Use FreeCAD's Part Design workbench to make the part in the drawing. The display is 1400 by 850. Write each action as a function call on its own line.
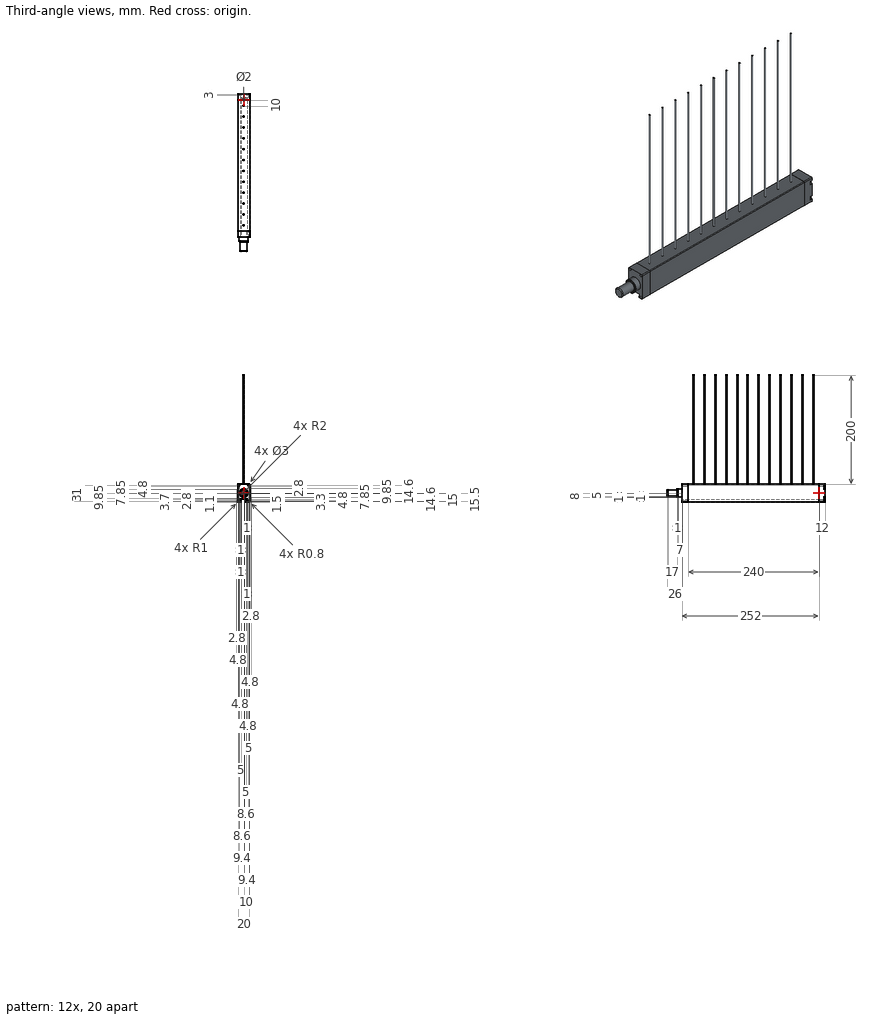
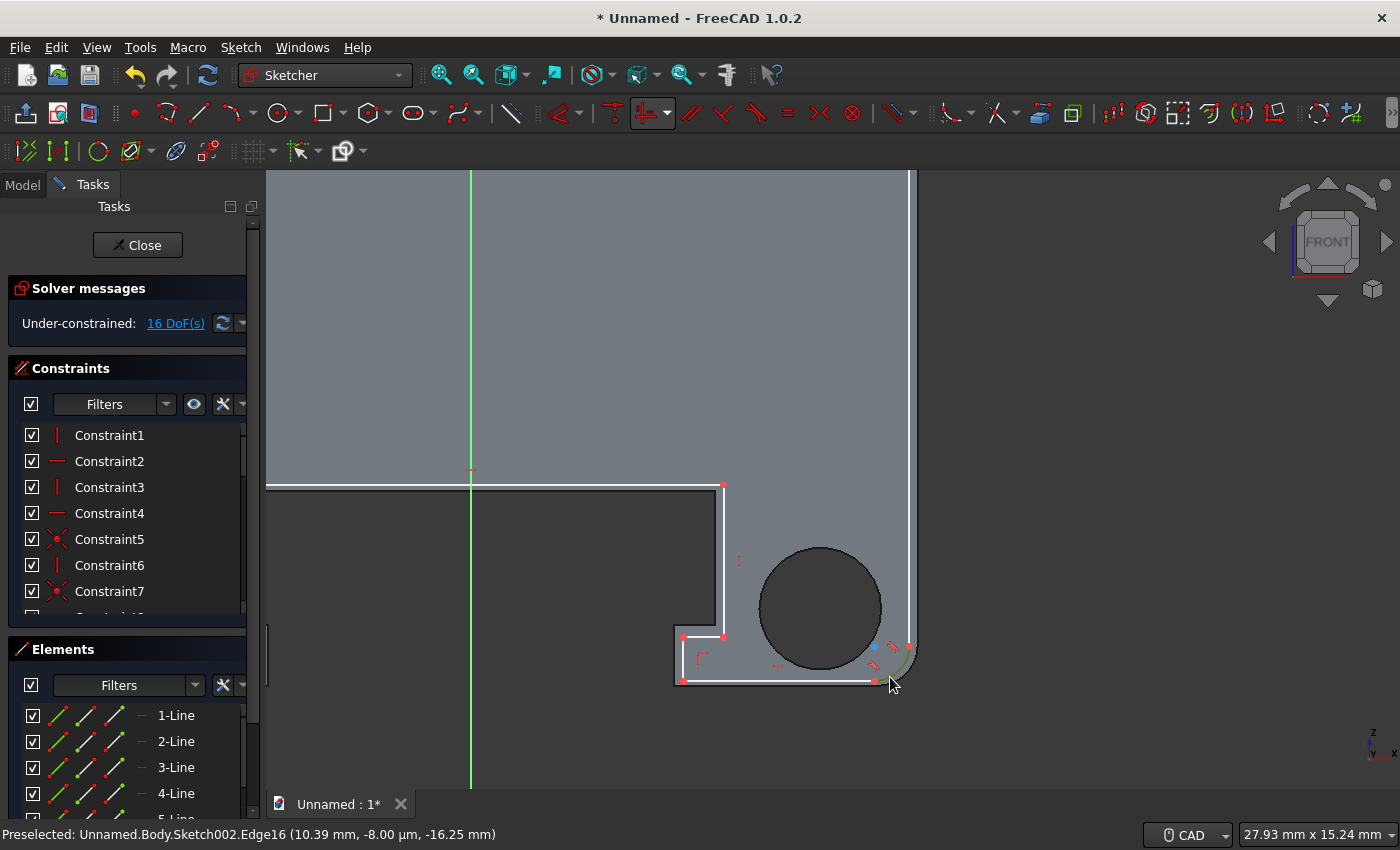
click(788, 114)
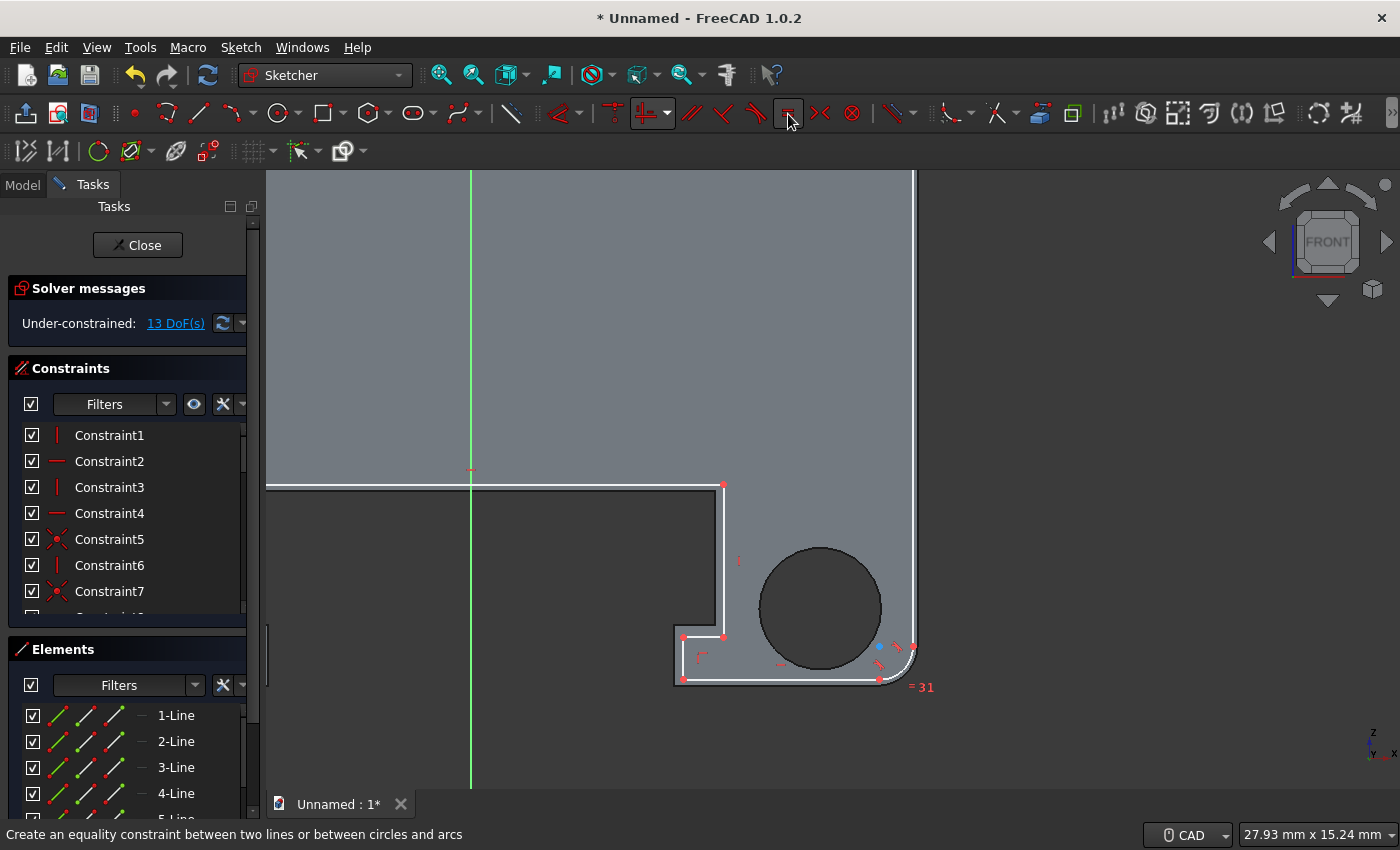
key(d)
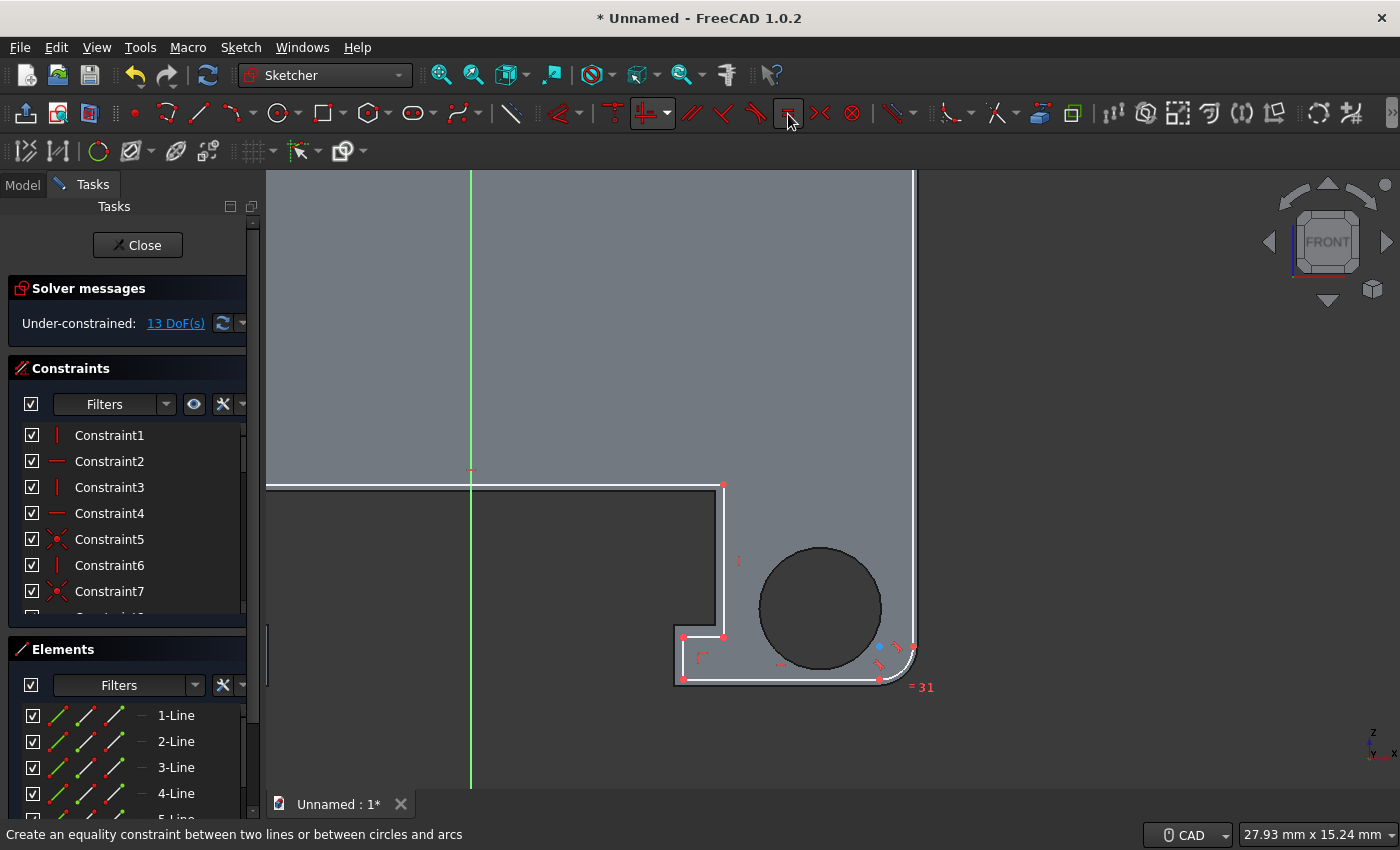
scroll(891, 679, down, 6)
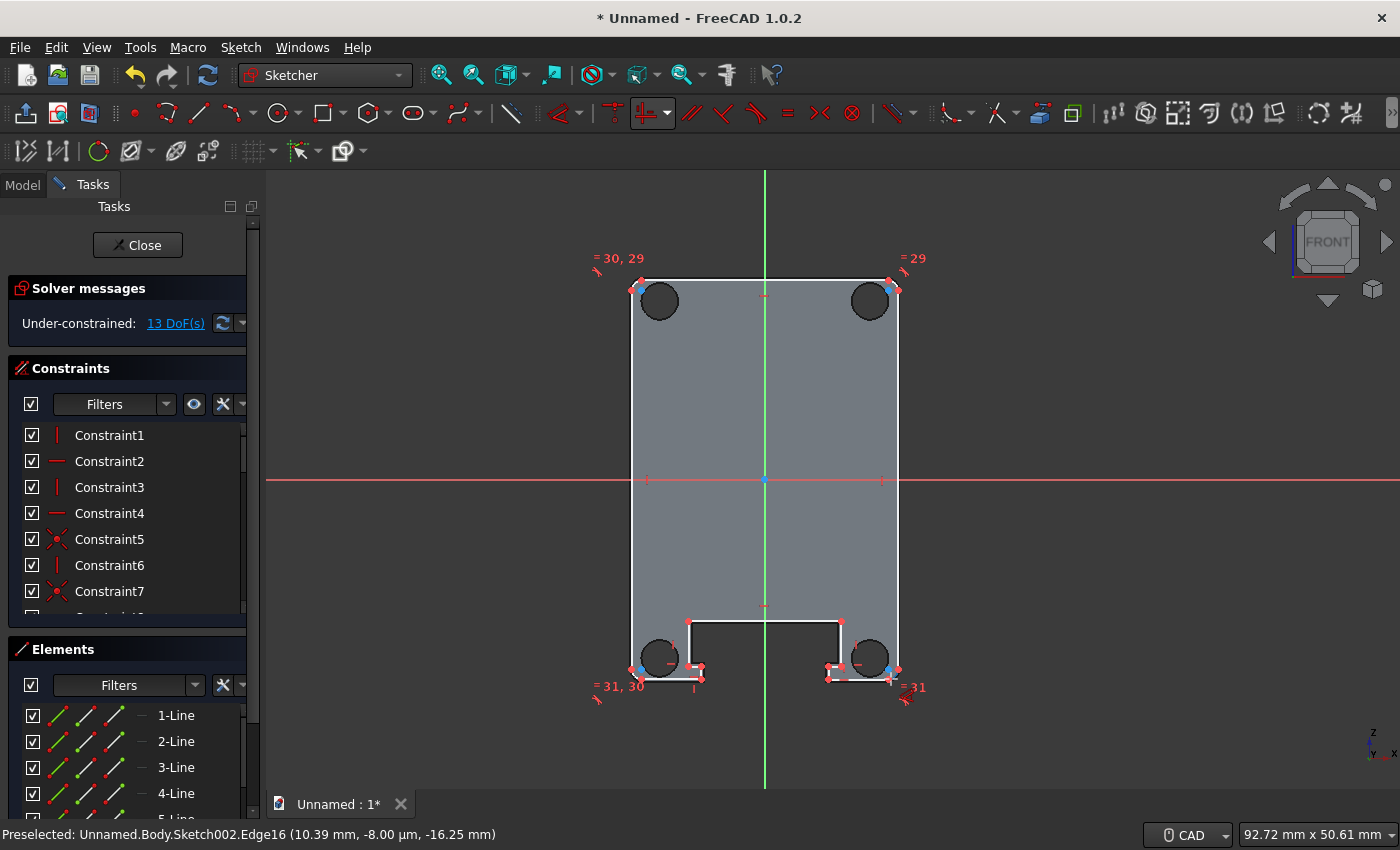
scroll(897, 286, up, 8)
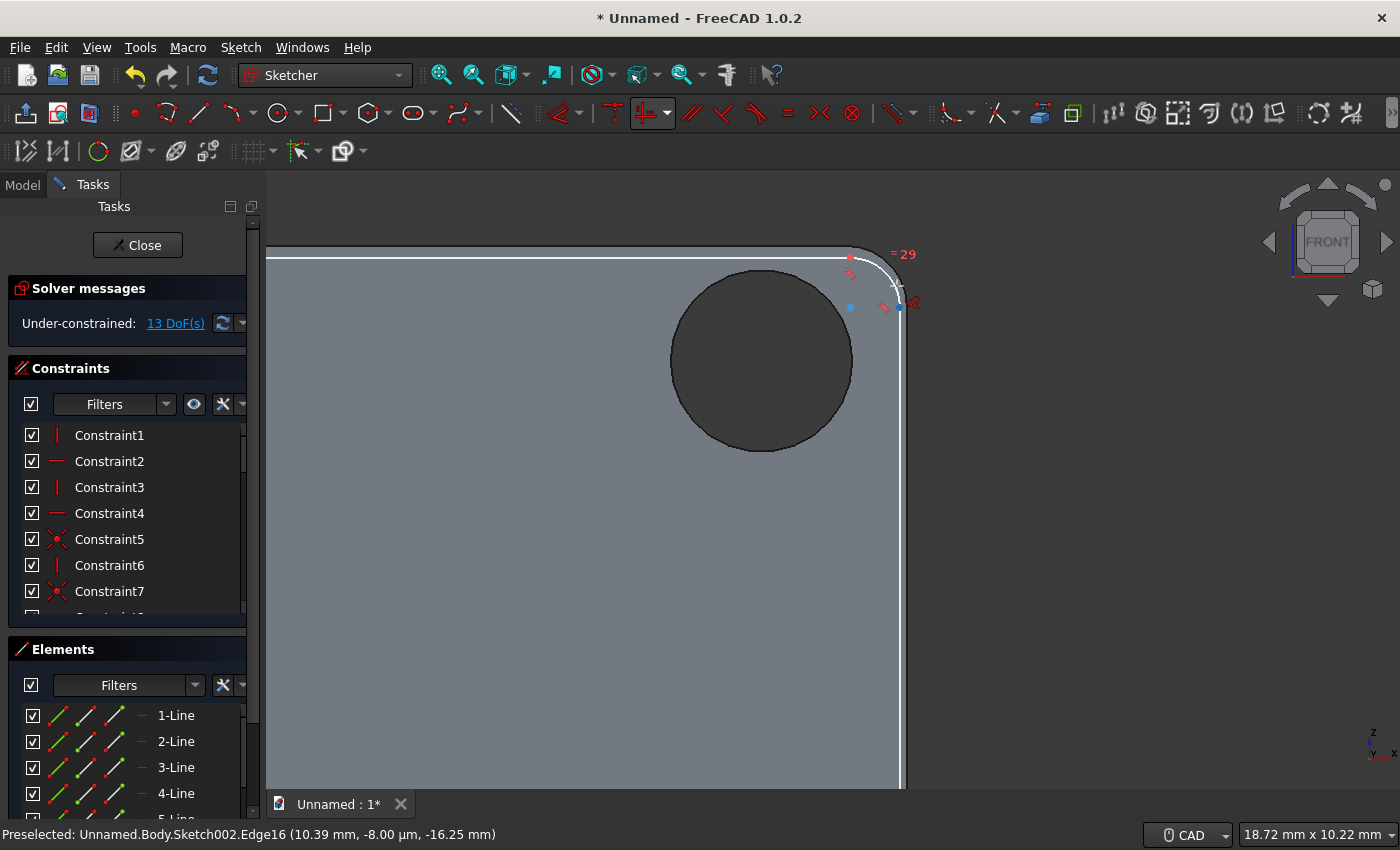
click(894, 285)
click(922, 270)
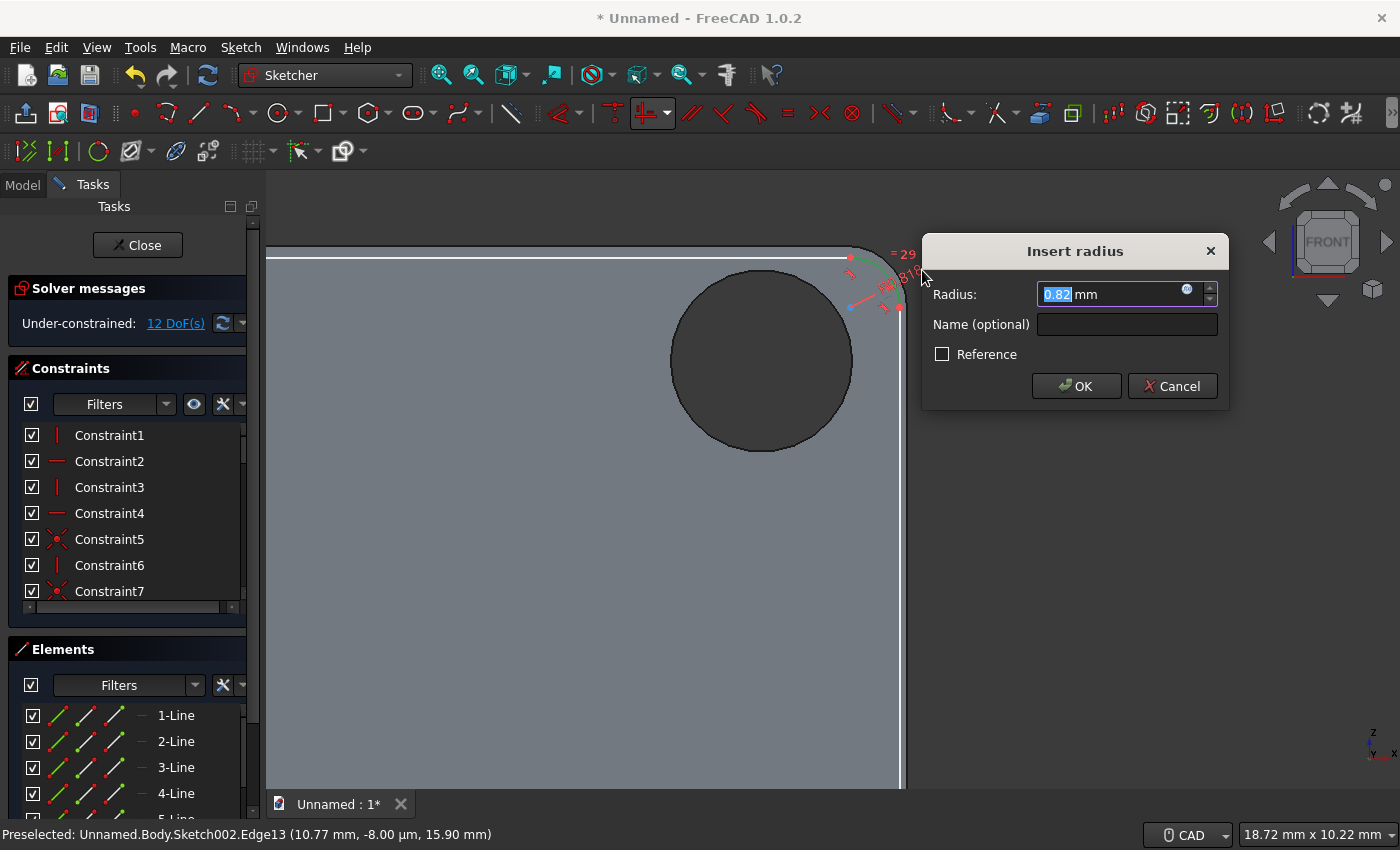
text(0.8)
key(Return)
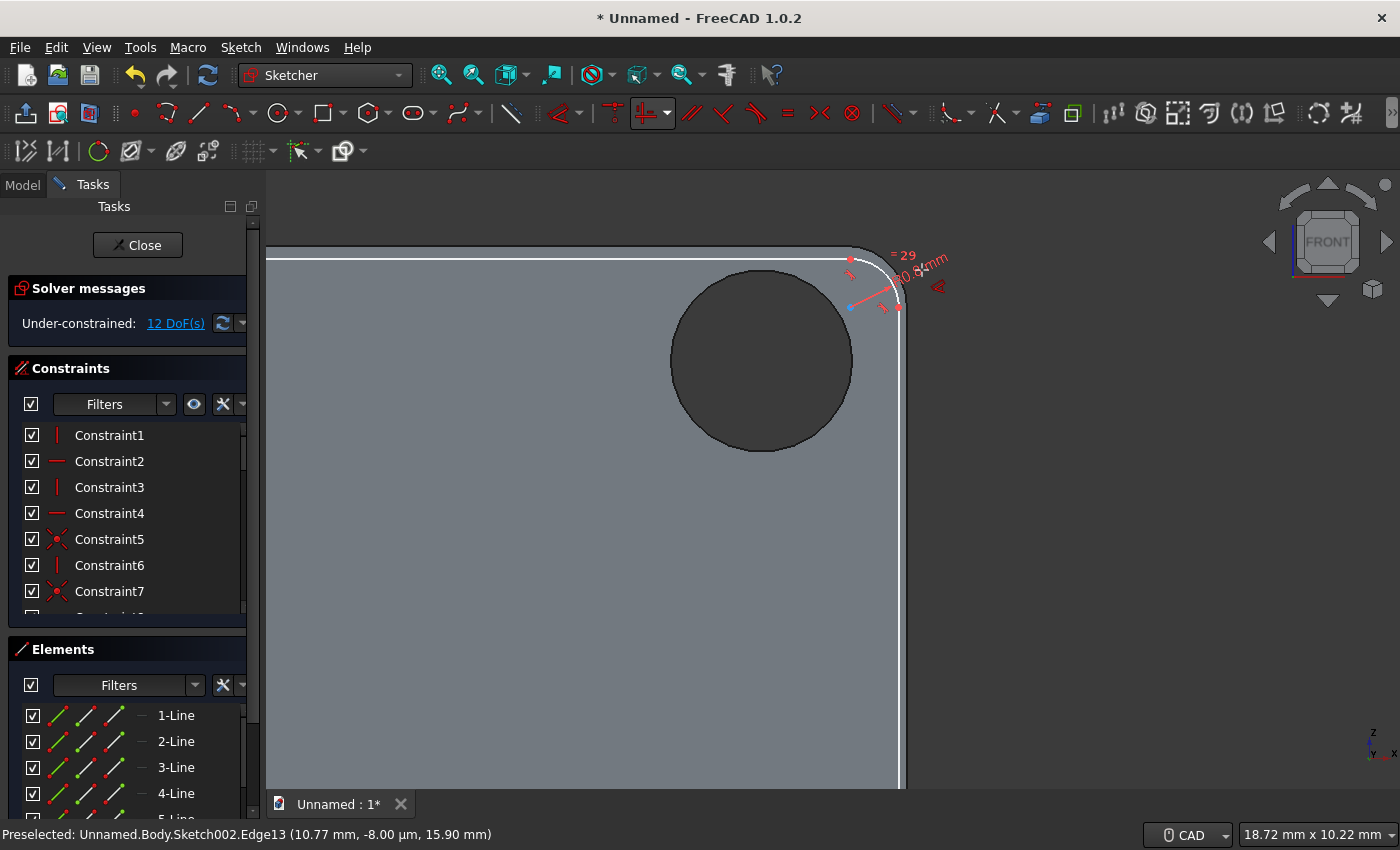
scroll(897, 286, down, 8)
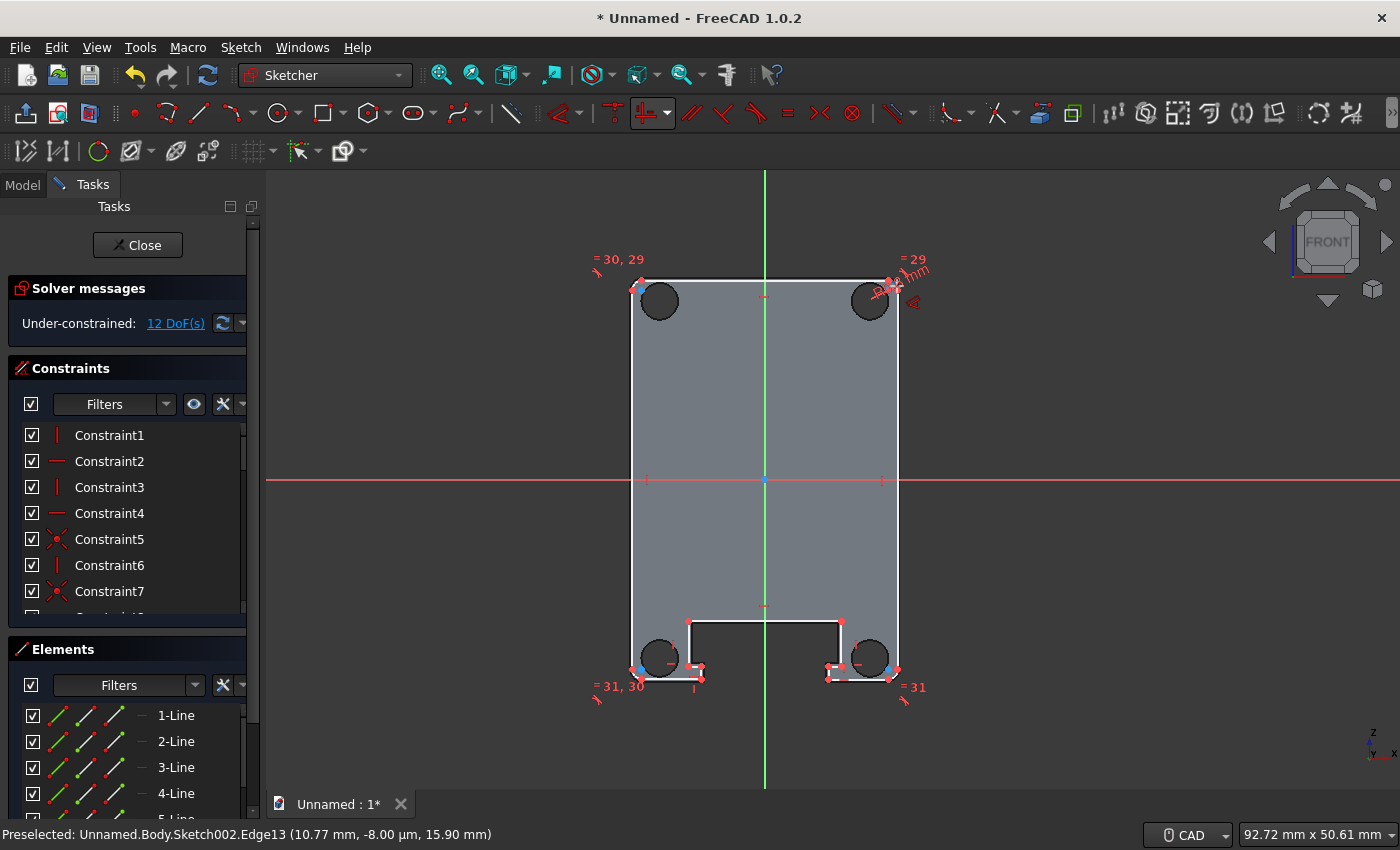
scroll(697, 667, up, 7)